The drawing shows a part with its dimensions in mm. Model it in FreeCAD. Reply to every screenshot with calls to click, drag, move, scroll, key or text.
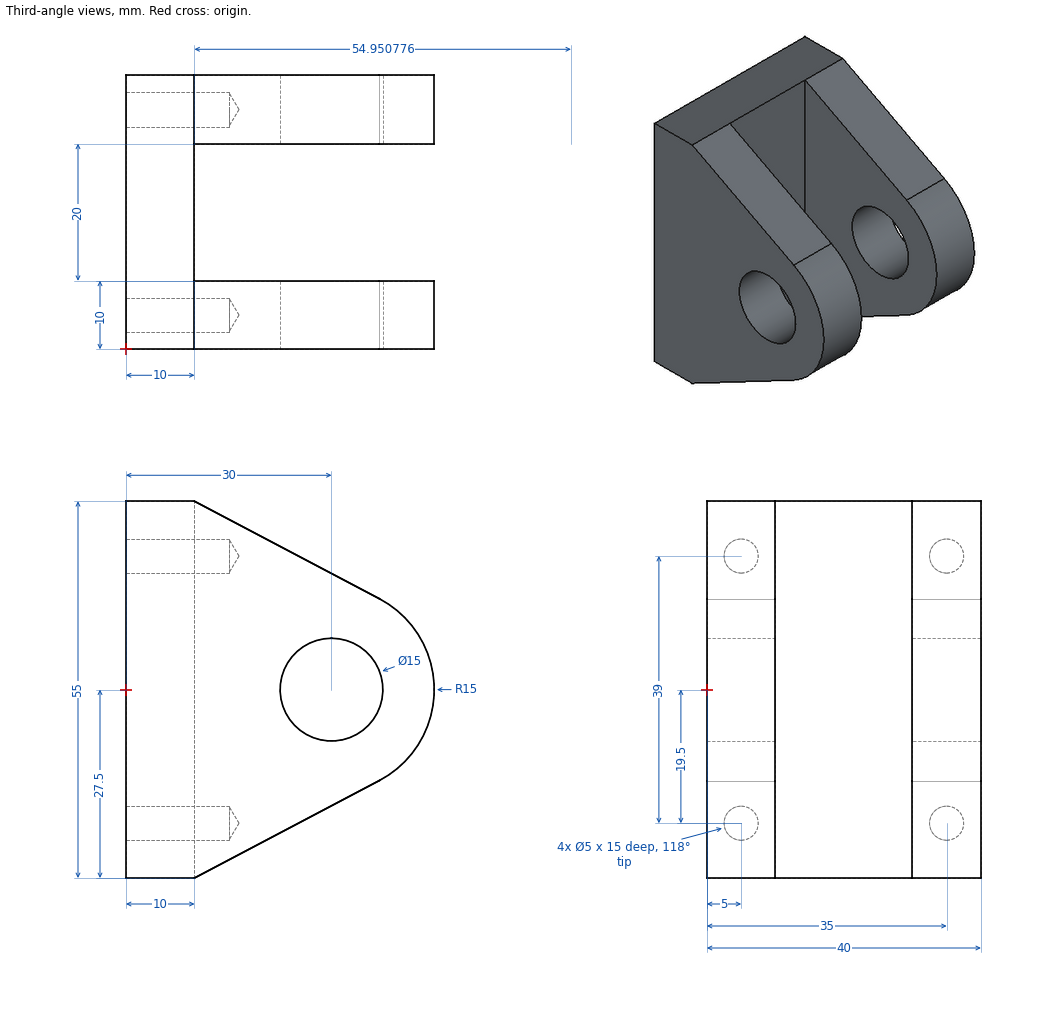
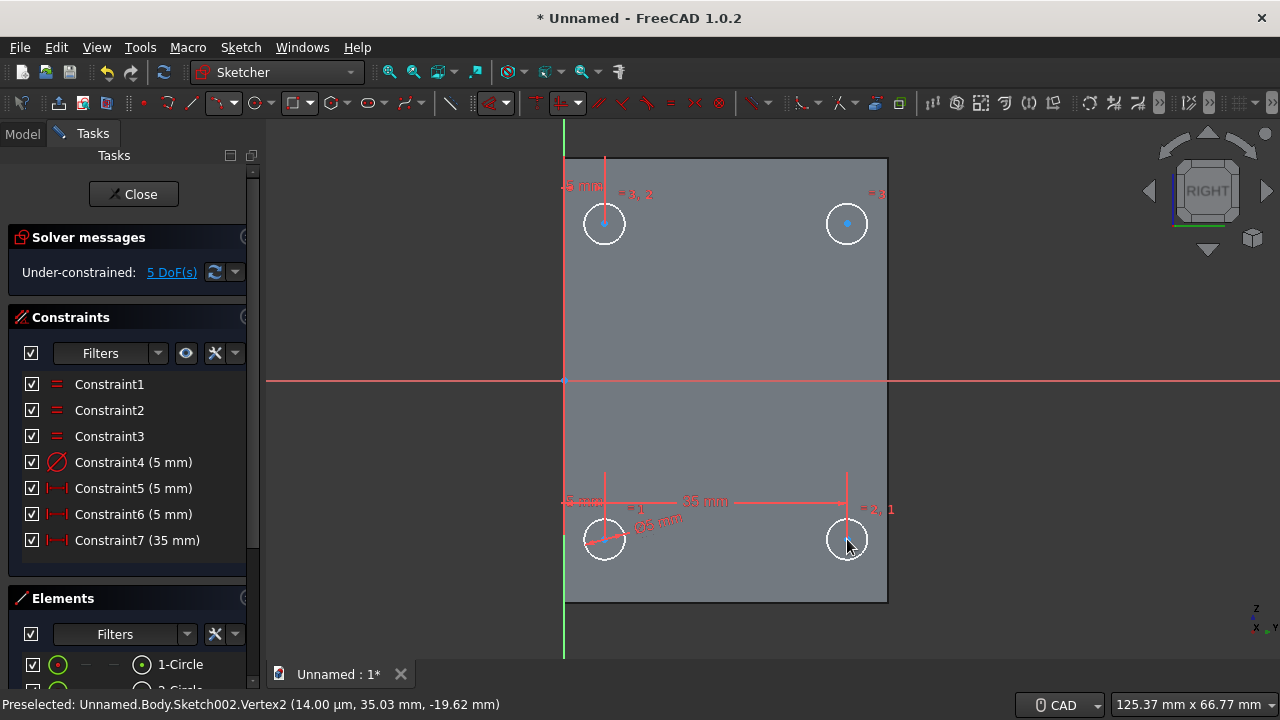
click(847, 224)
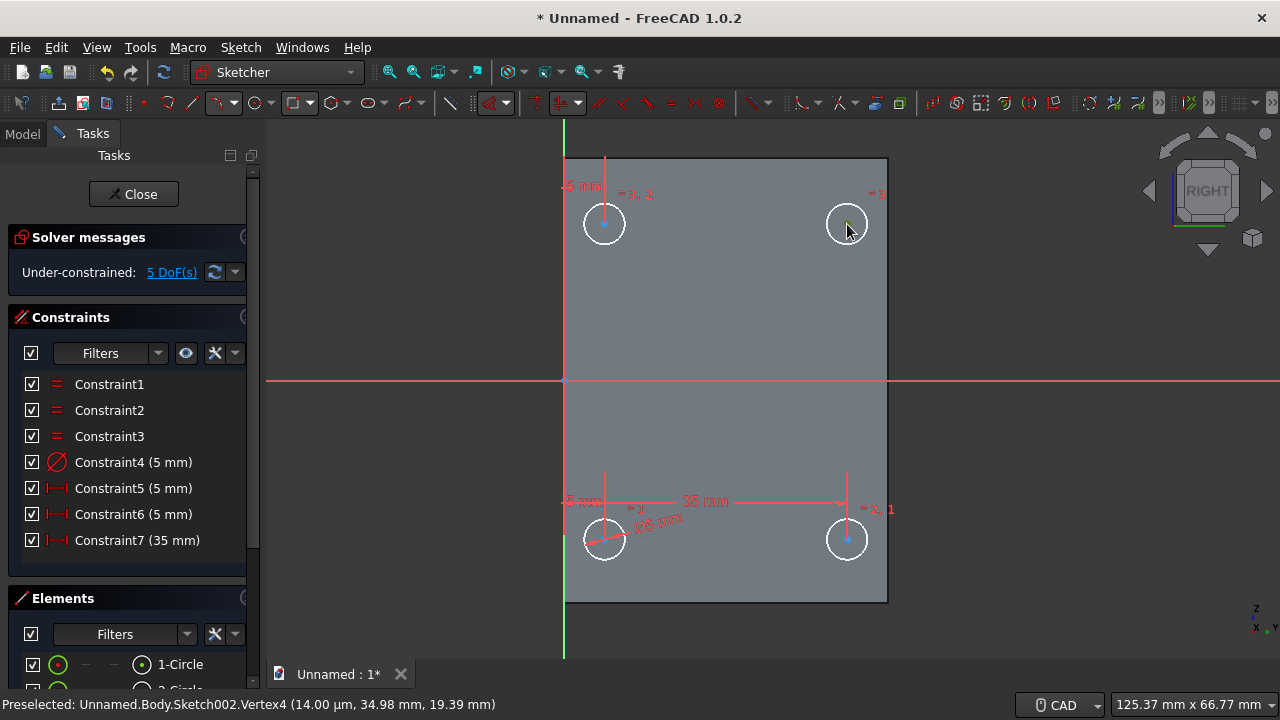
key(l)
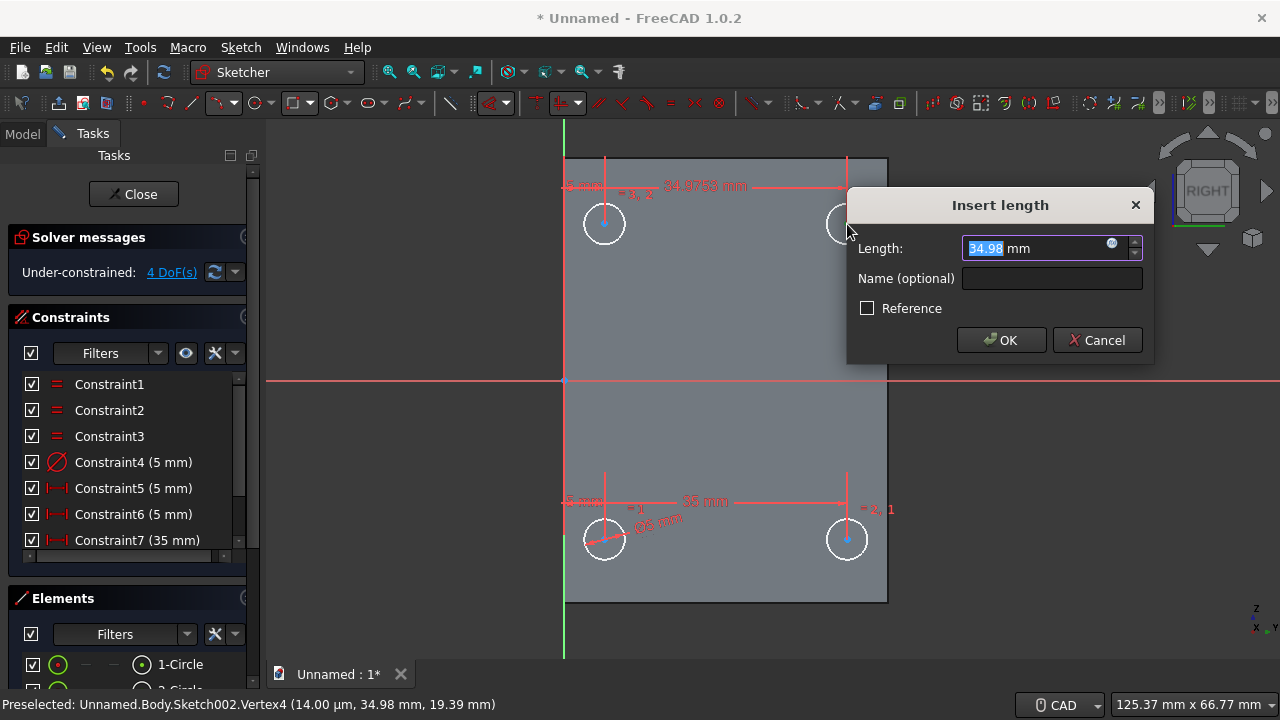
text(35)
key(Return)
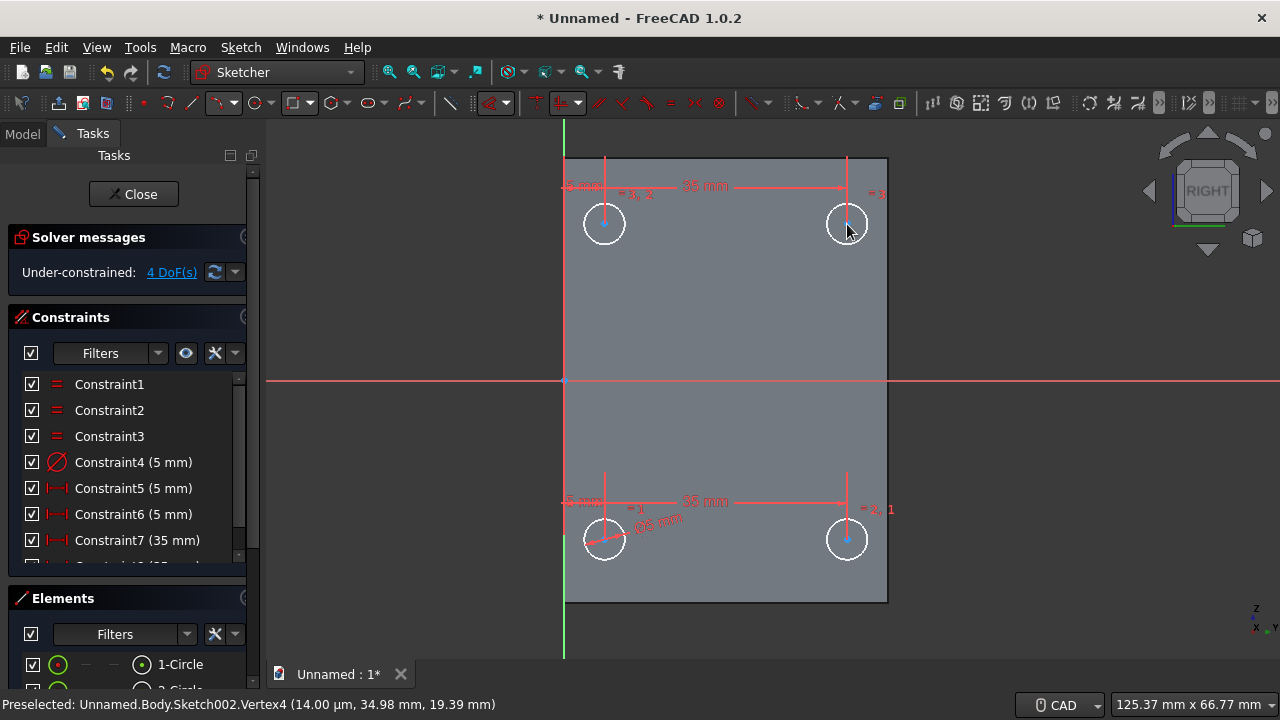
click(605, 539)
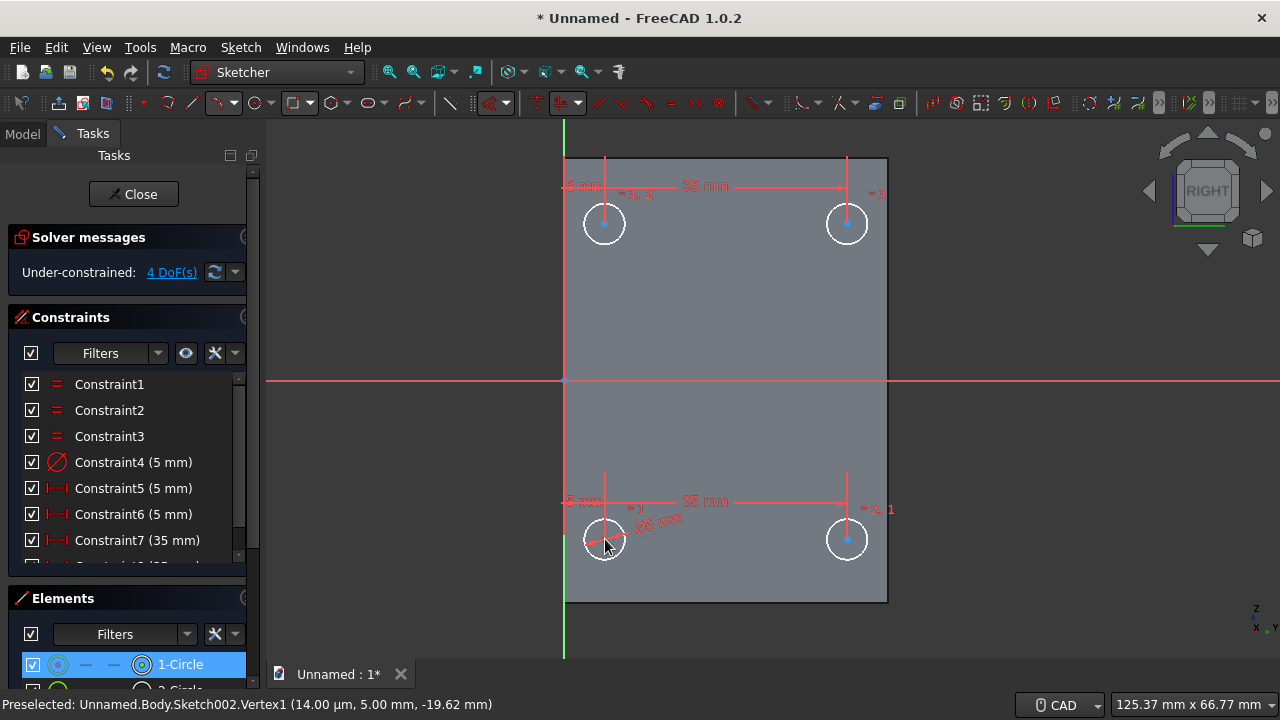
click(605, 224)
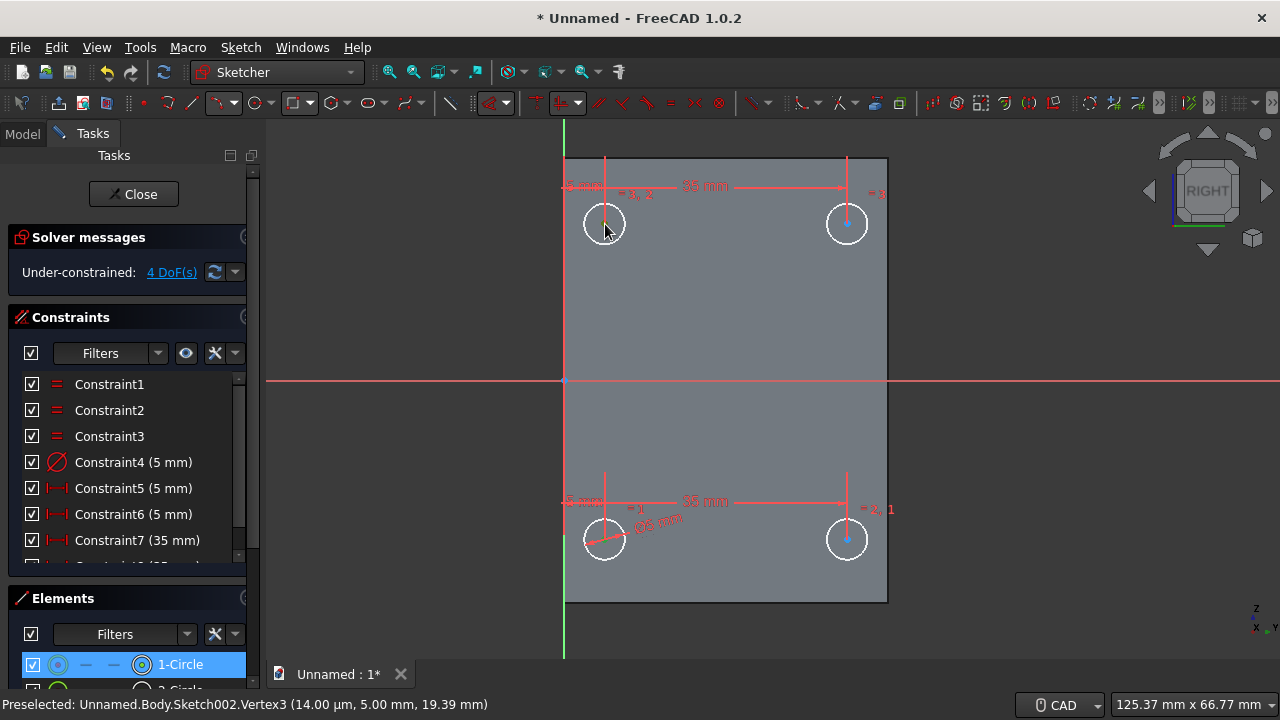
key(i)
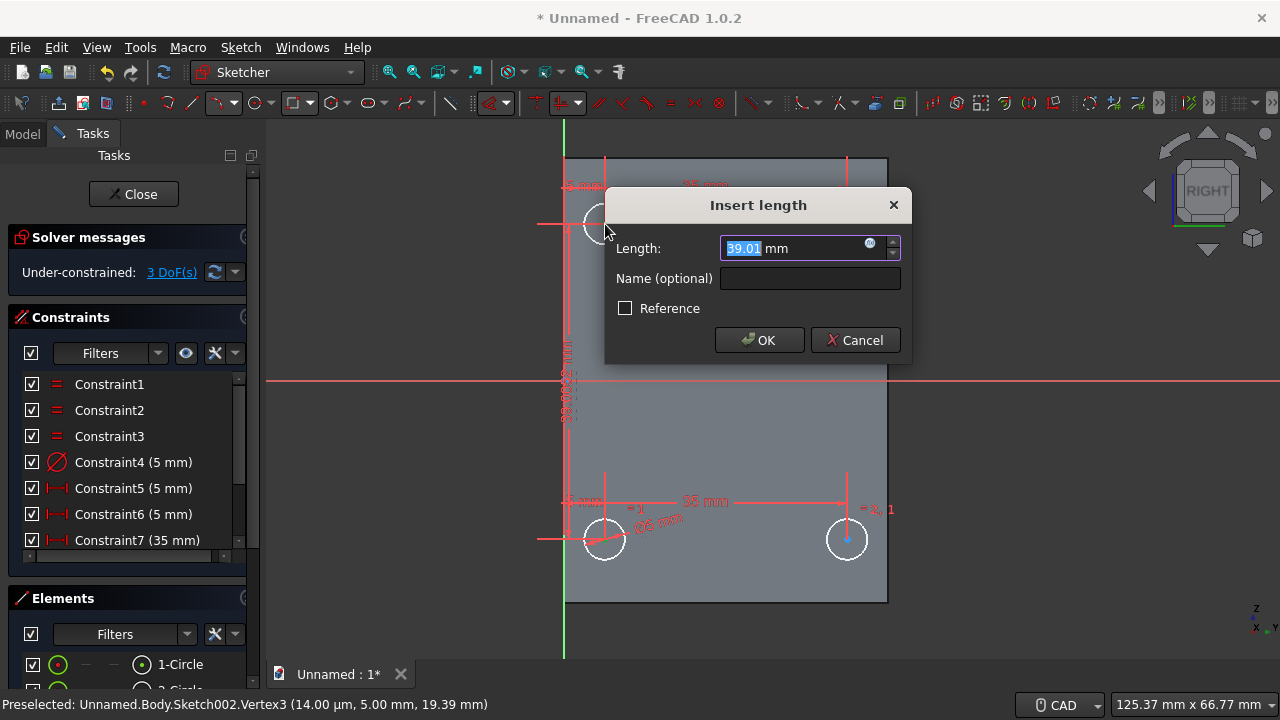
text(39)
key(Return)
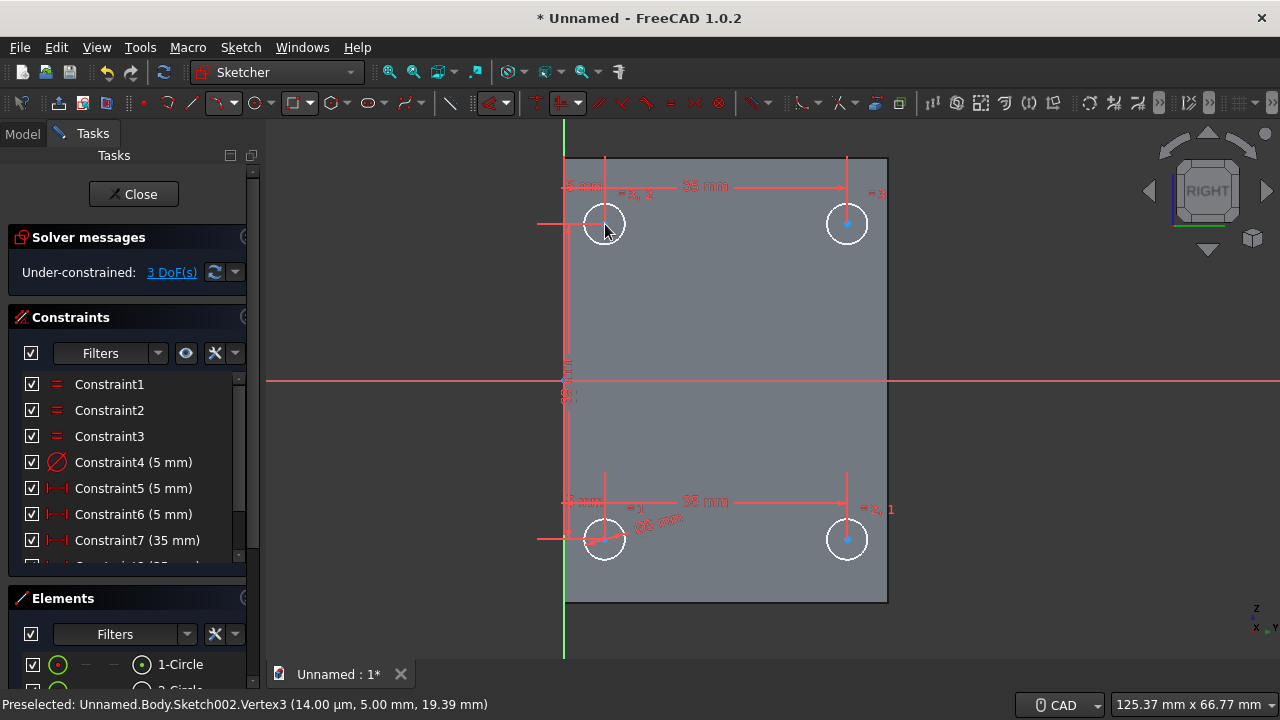
click(847, 539)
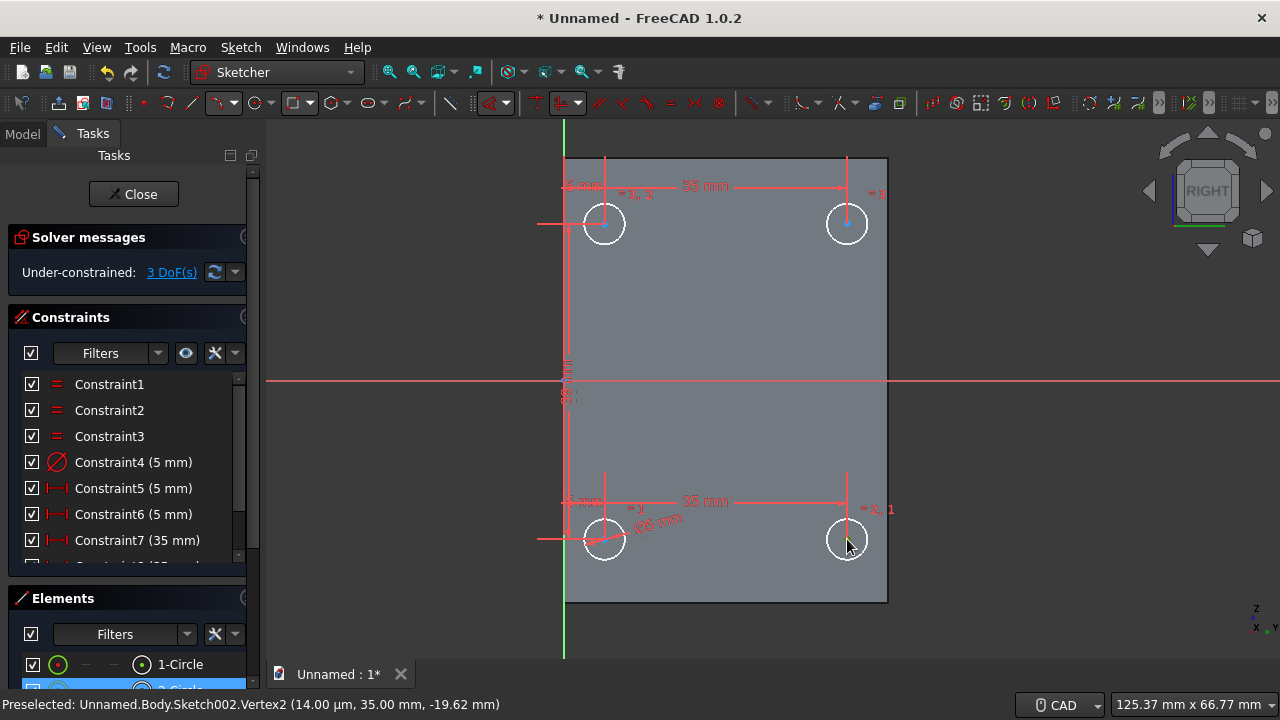
click(605, 224)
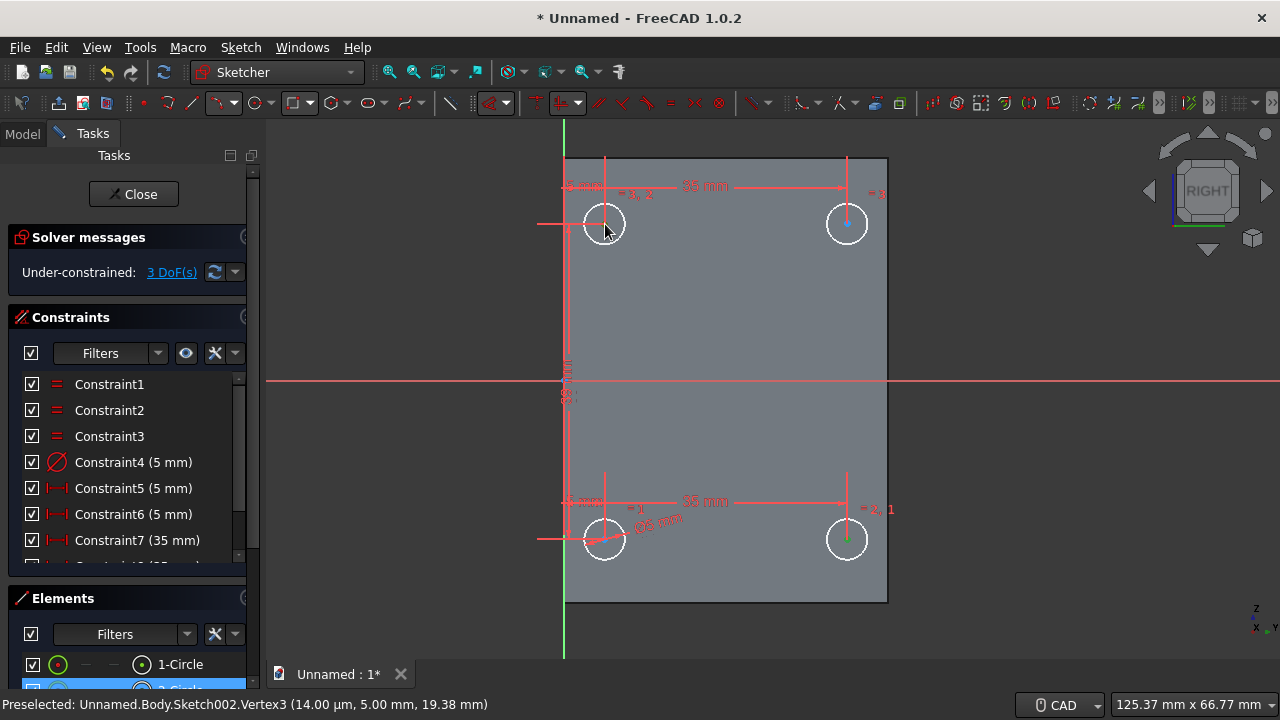
key(i)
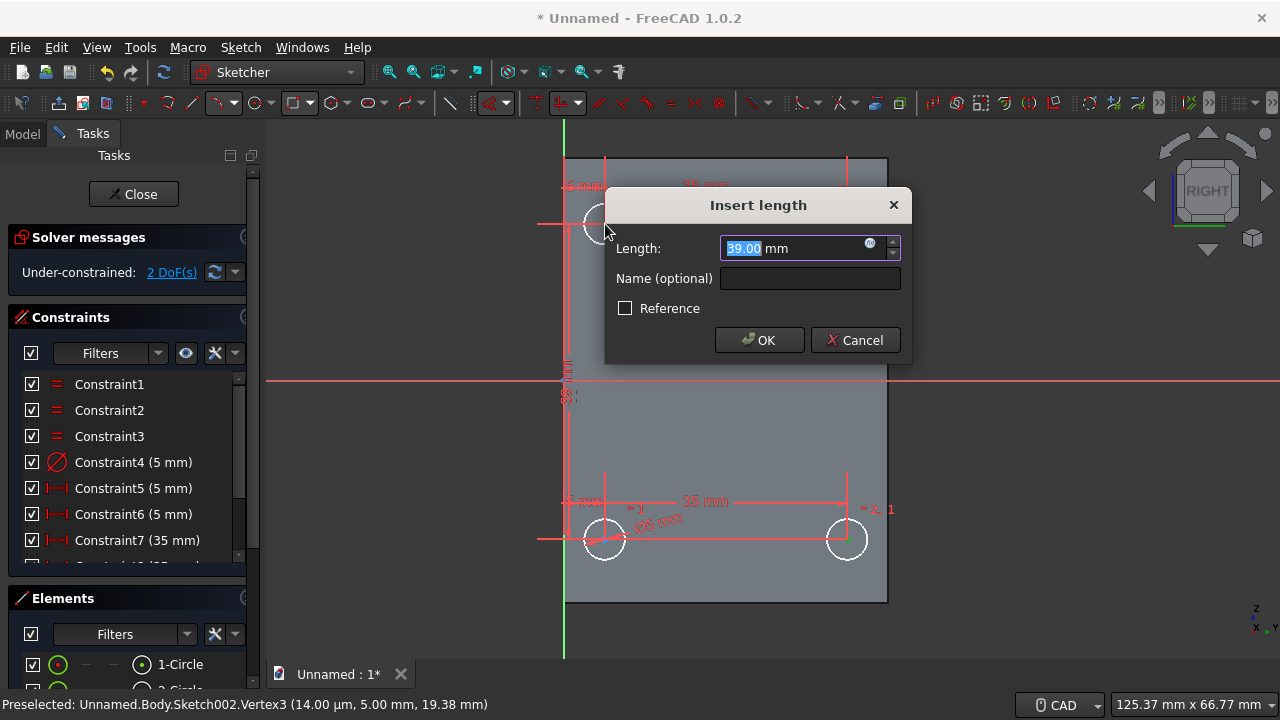
text(39)
key(Return)